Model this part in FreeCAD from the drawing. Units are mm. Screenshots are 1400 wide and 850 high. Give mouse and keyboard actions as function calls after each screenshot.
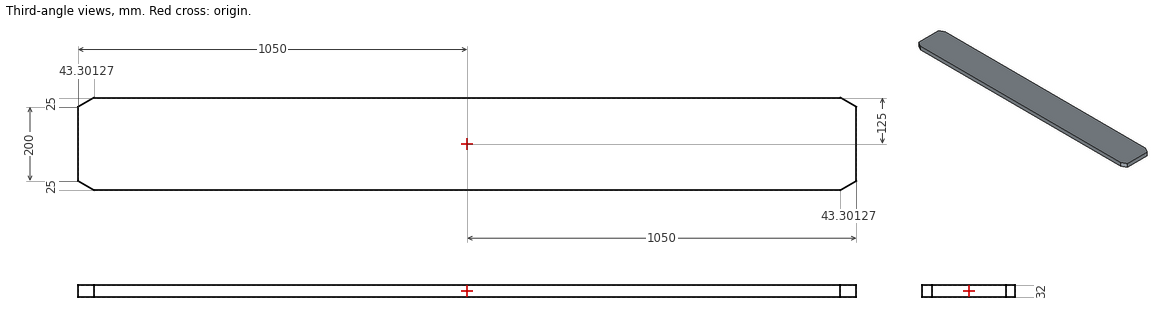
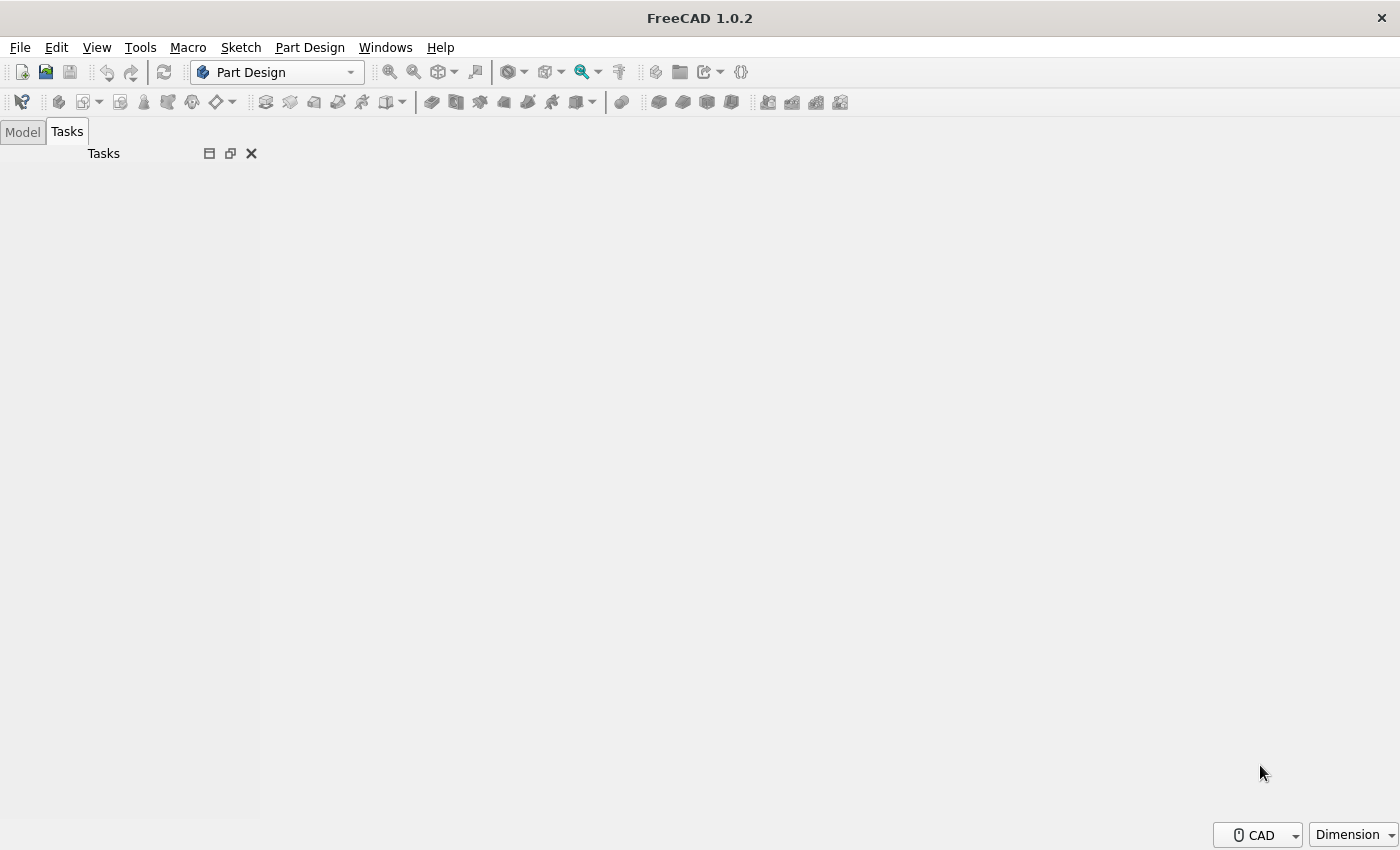
click(22, 72)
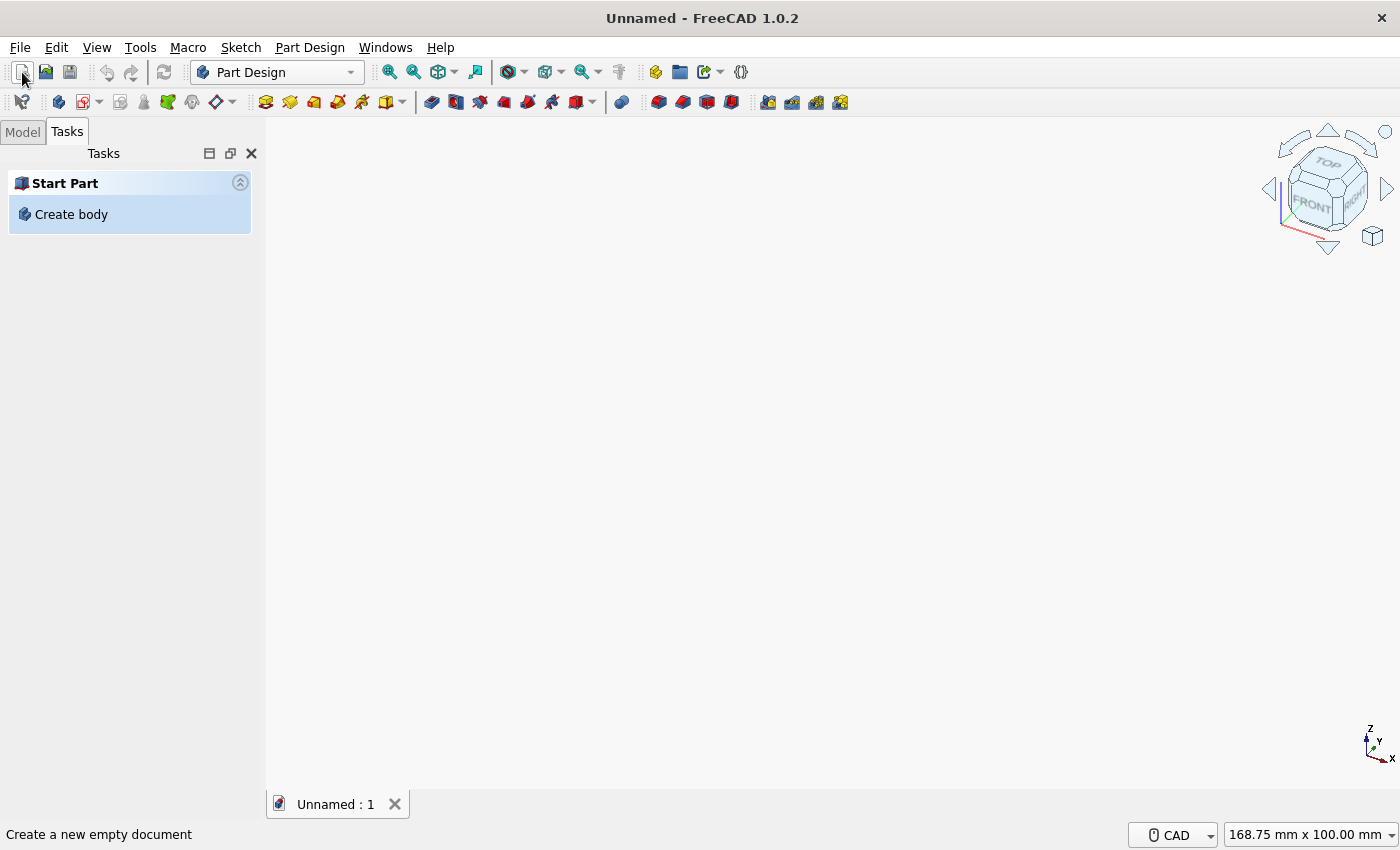
click(84, 102)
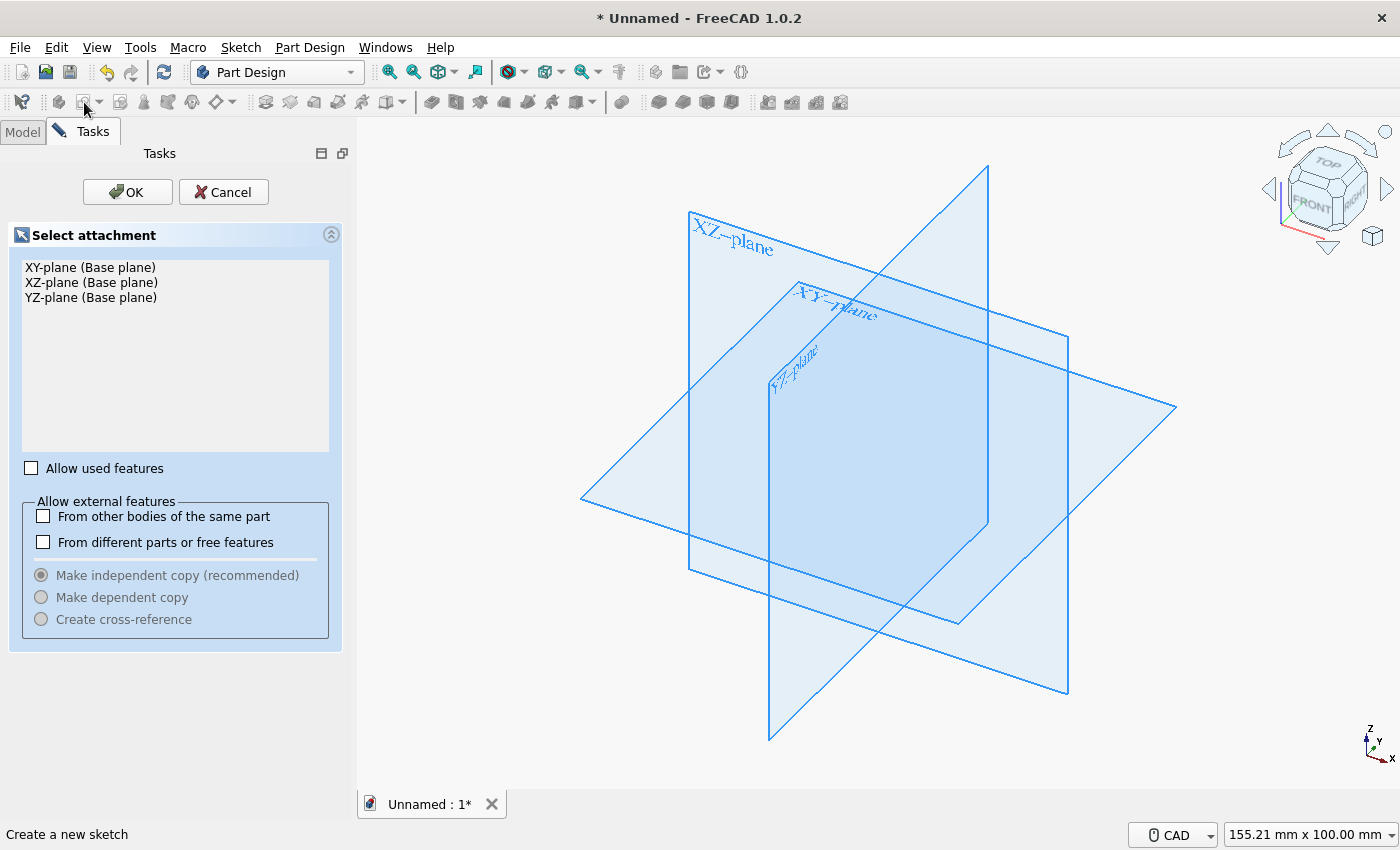
click(82, 268)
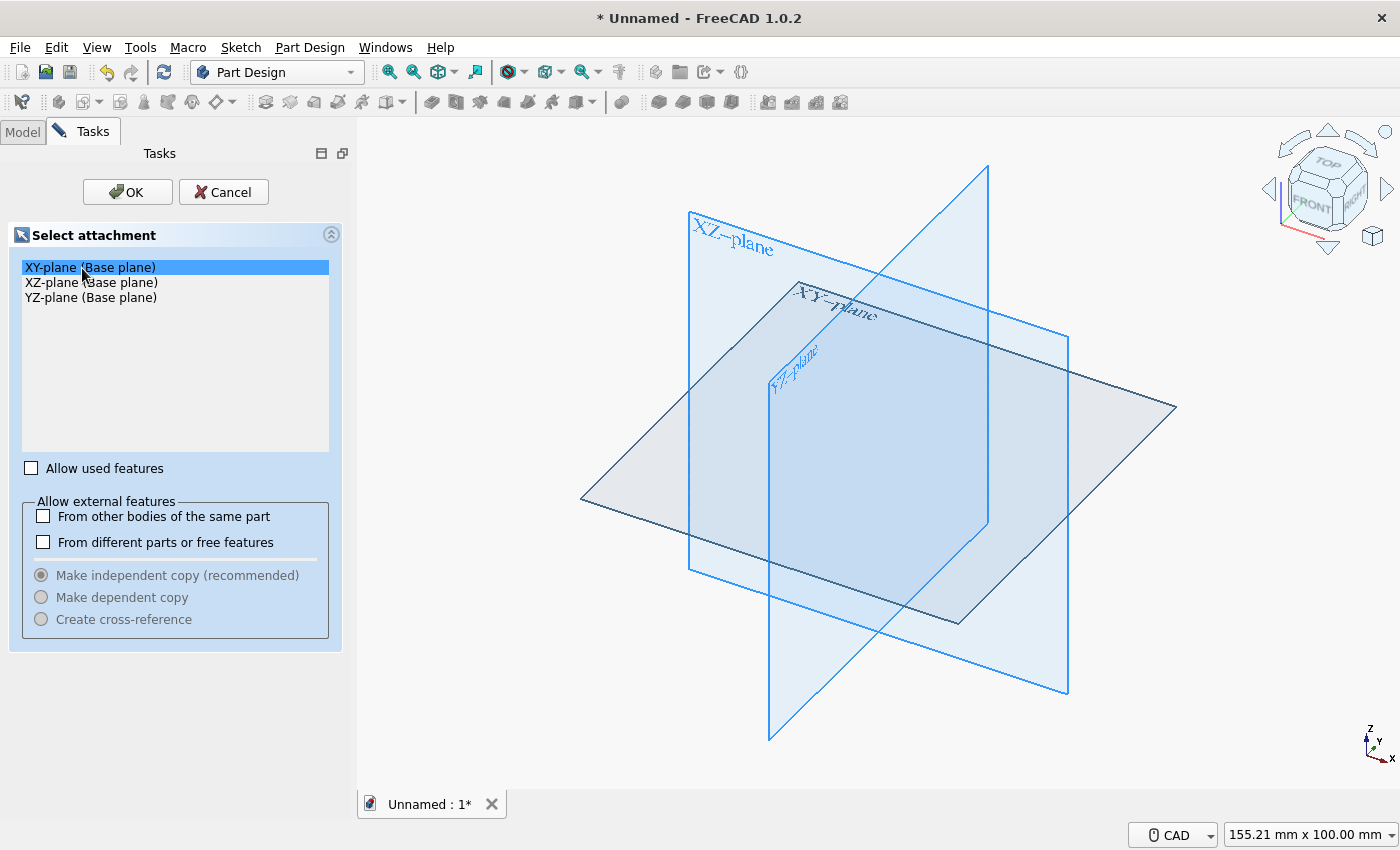
click(128, 192)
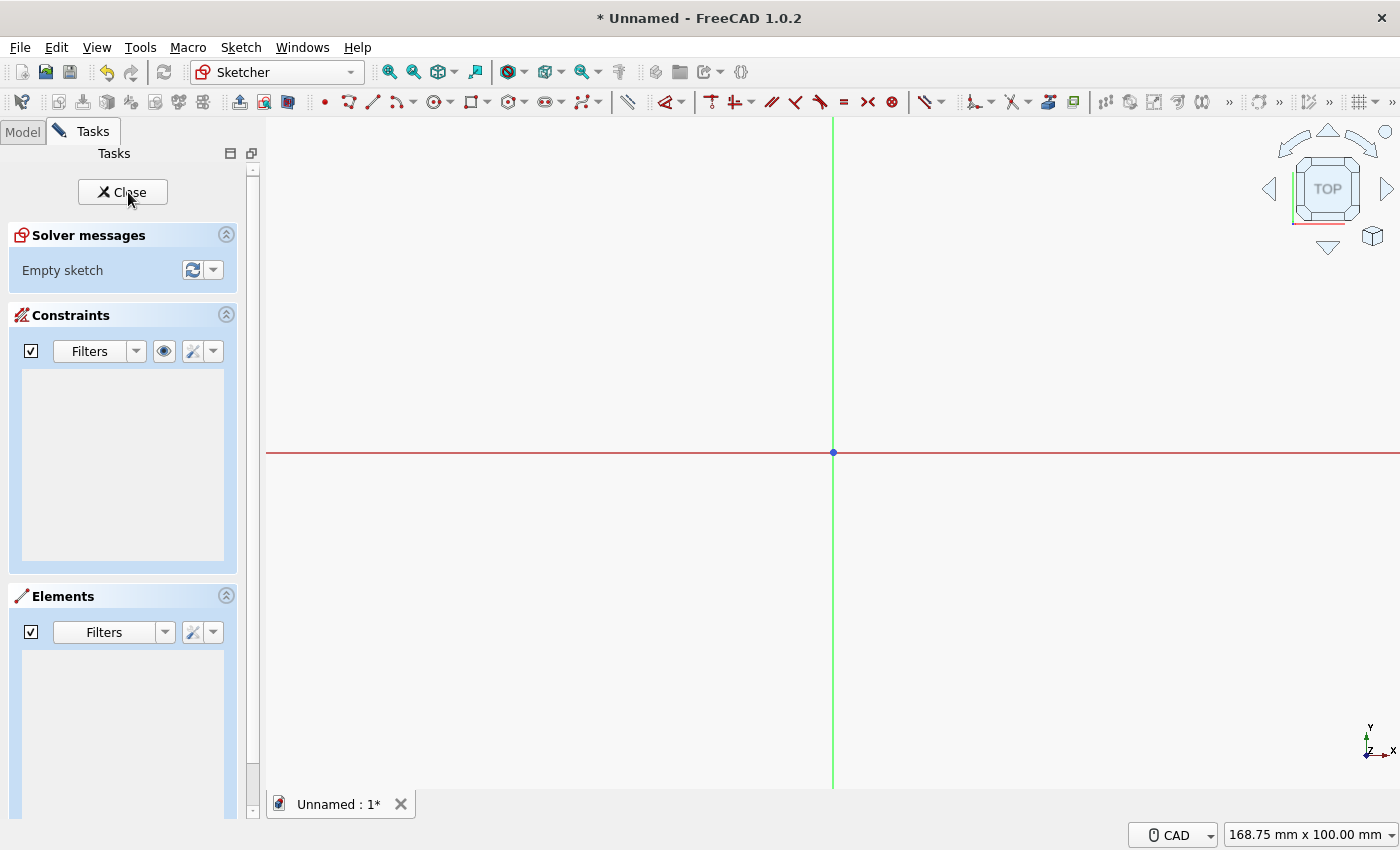
scroll(761, 453, down, 15)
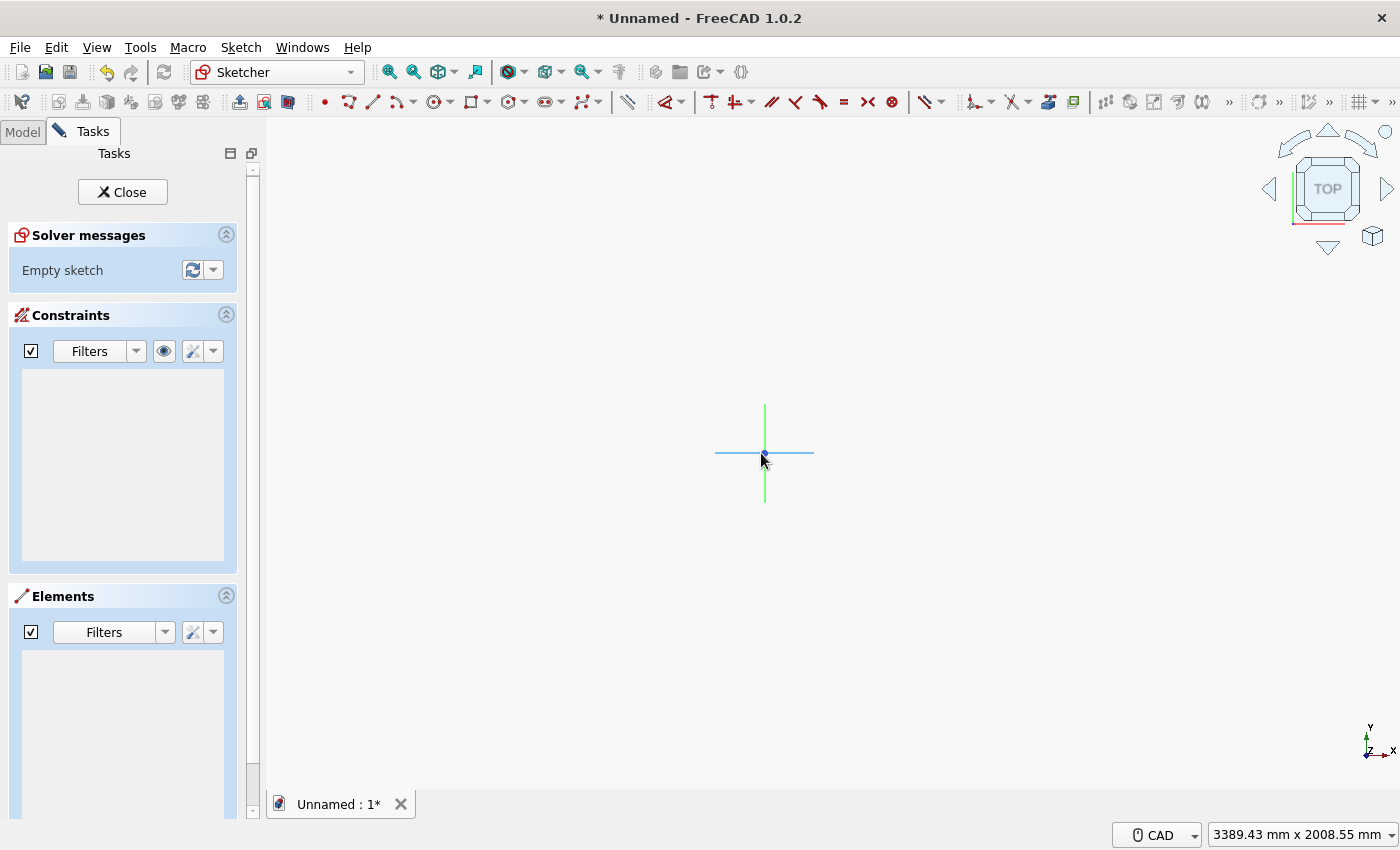
click(350, 102)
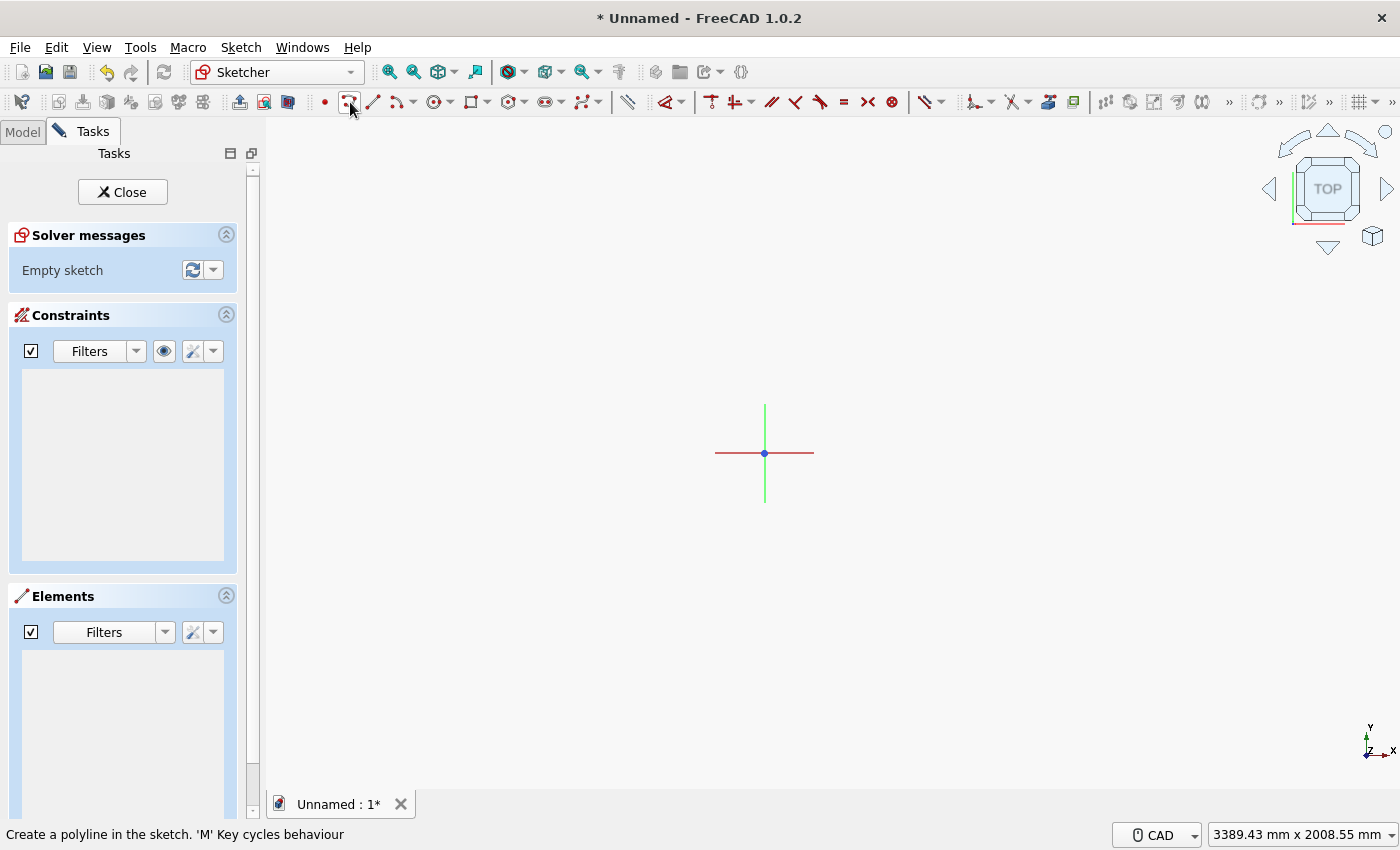
click(1102, 412)
click(428, 412)
click(414, 420)
click(414, 487)
click(428, 495)
click(1102, 495)
click(1116, 487)
click(1116, 420)
click(1102, 413)
key(Escape)
key(Escape)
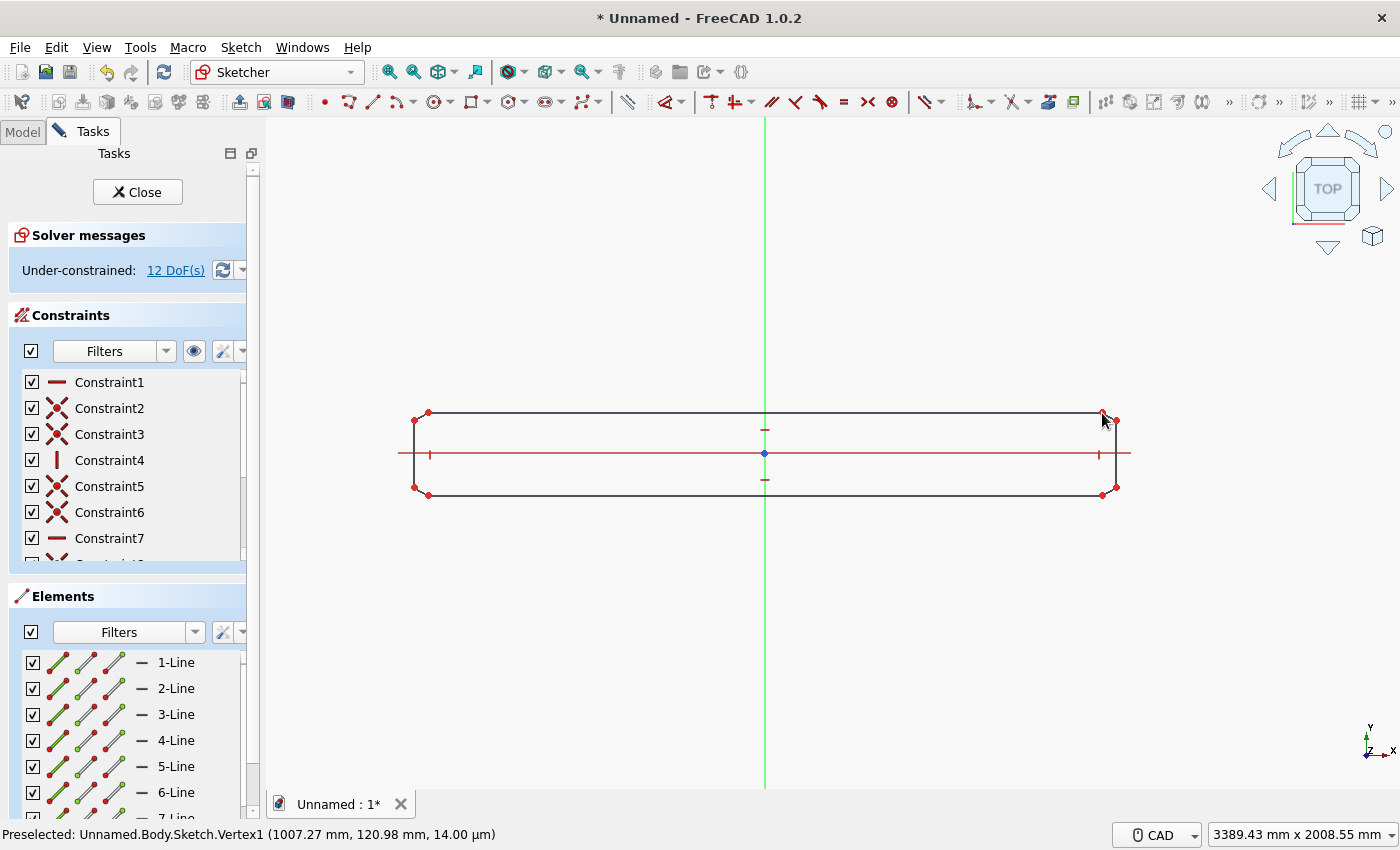
click(414, 441)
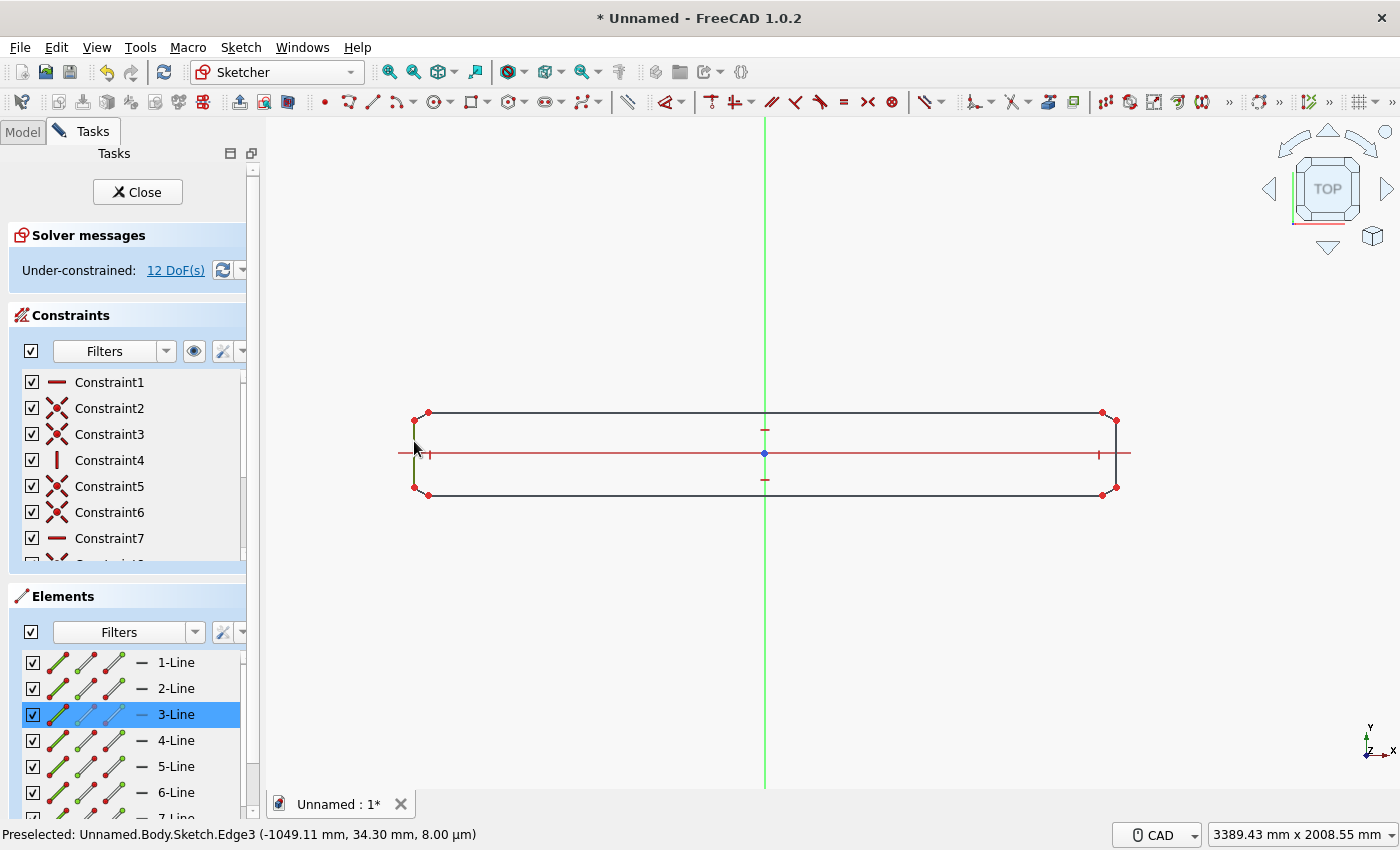
key(i)